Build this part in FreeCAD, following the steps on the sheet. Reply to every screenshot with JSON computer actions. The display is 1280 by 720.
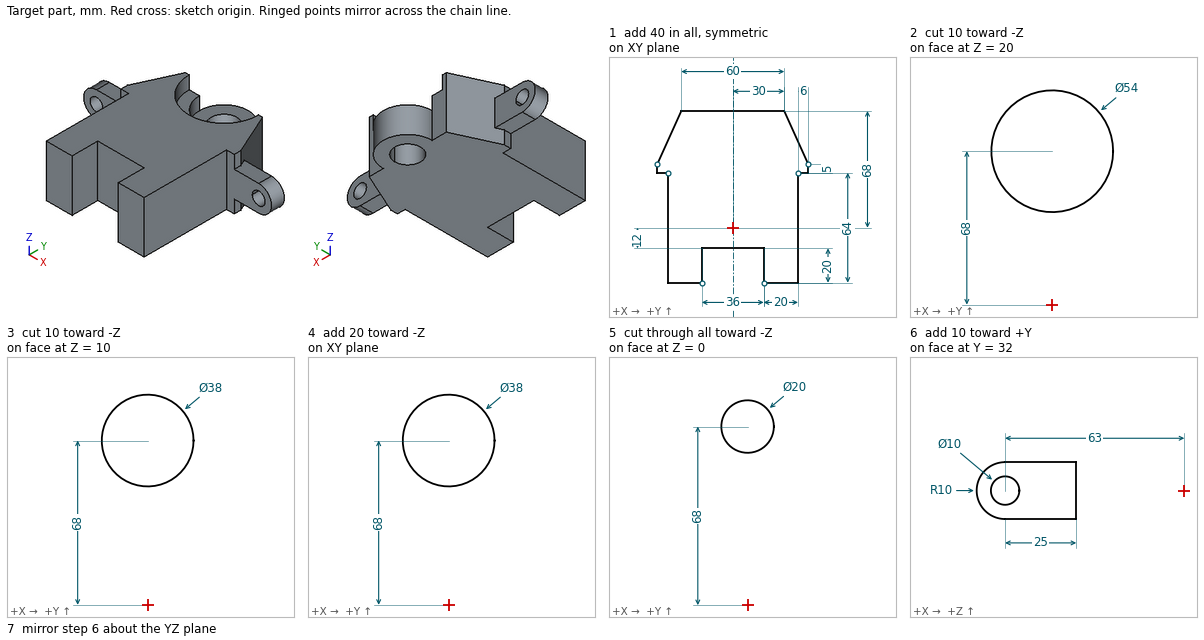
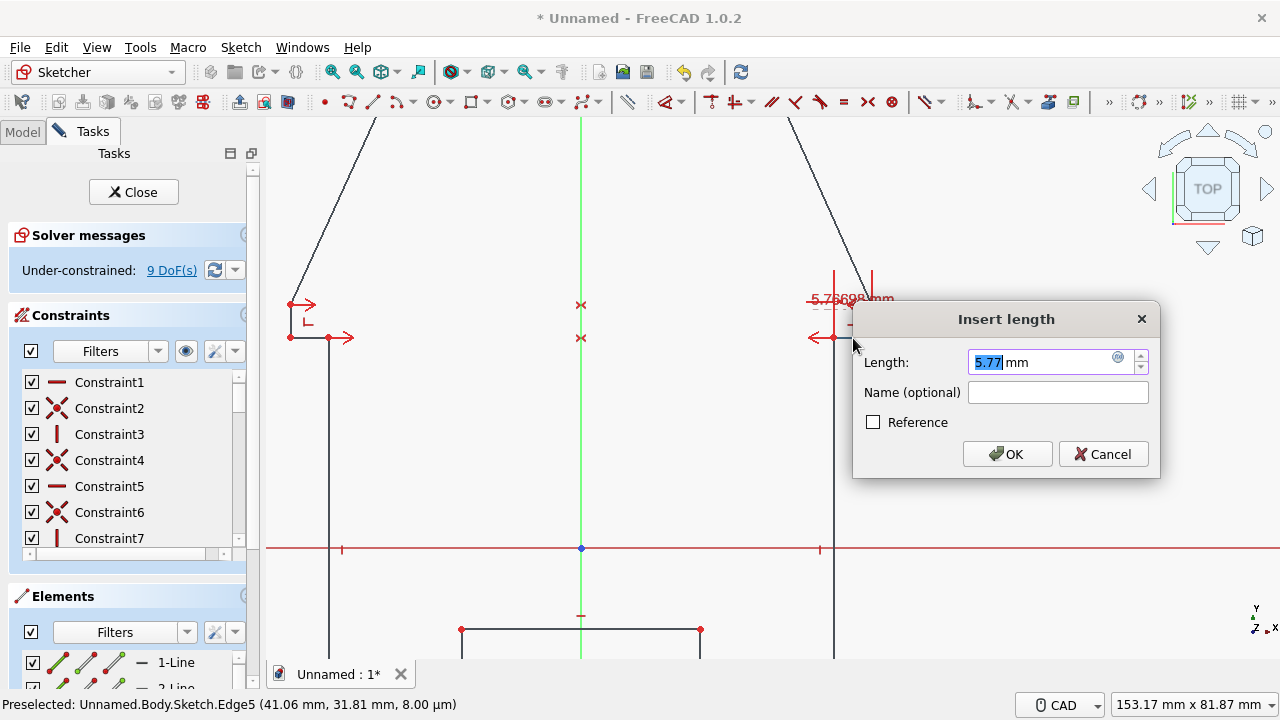
{"action": "type", "text": "6"}
{"action": "key", "text": "Return"}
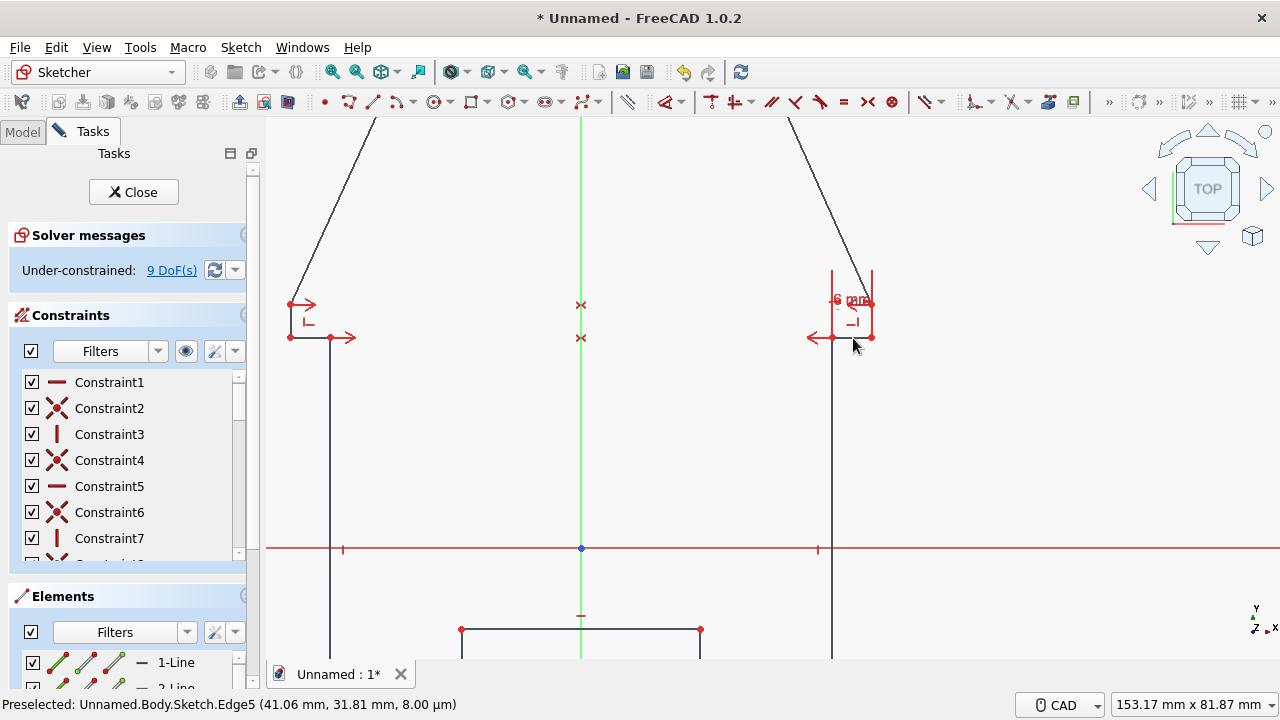
{"action": "scroll", "coordinate": [872, 328], "scroll_direction": "up", "scroll_amount": 2}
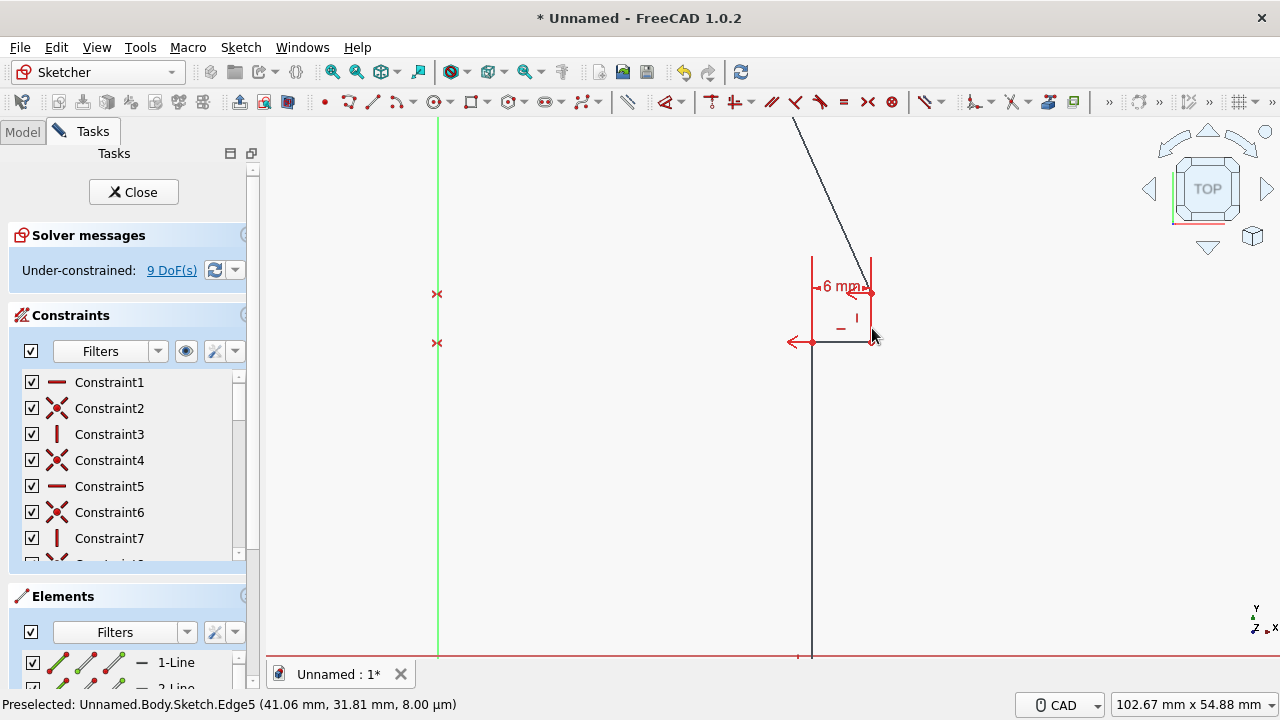
{"action": "left_click", "coordinate": [871, 328]}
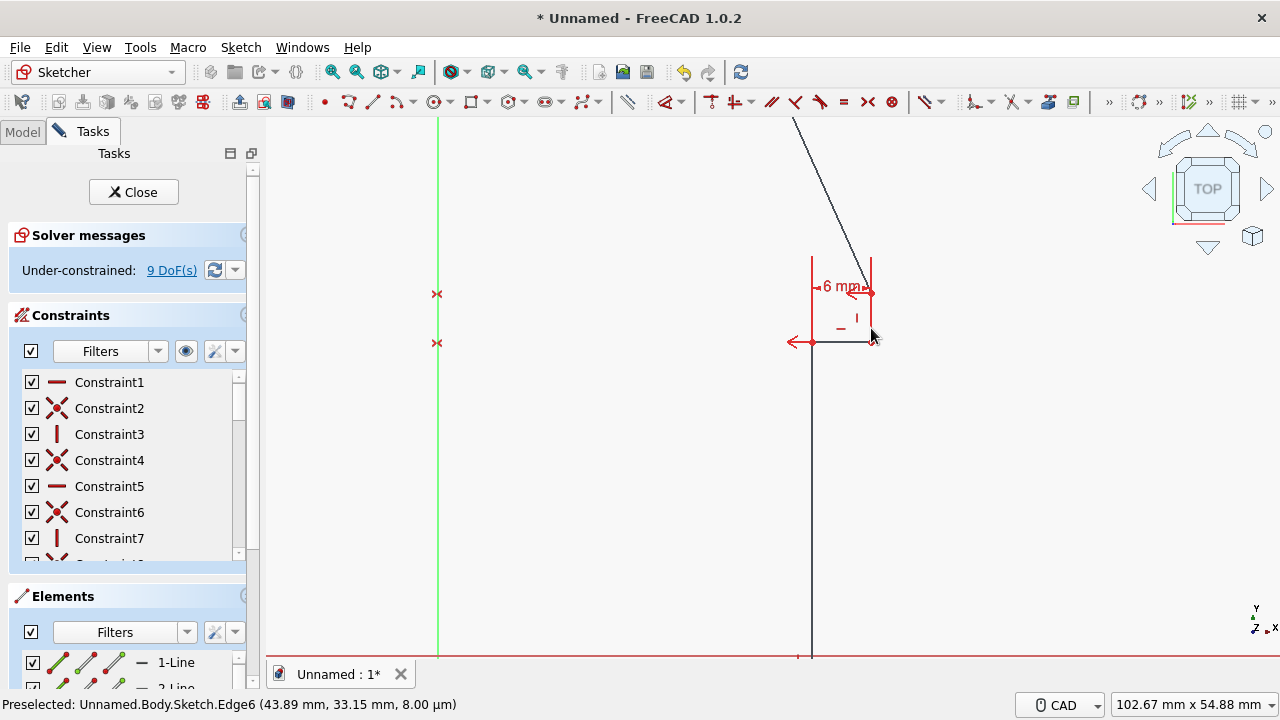
{"action": "key", "text": "i"}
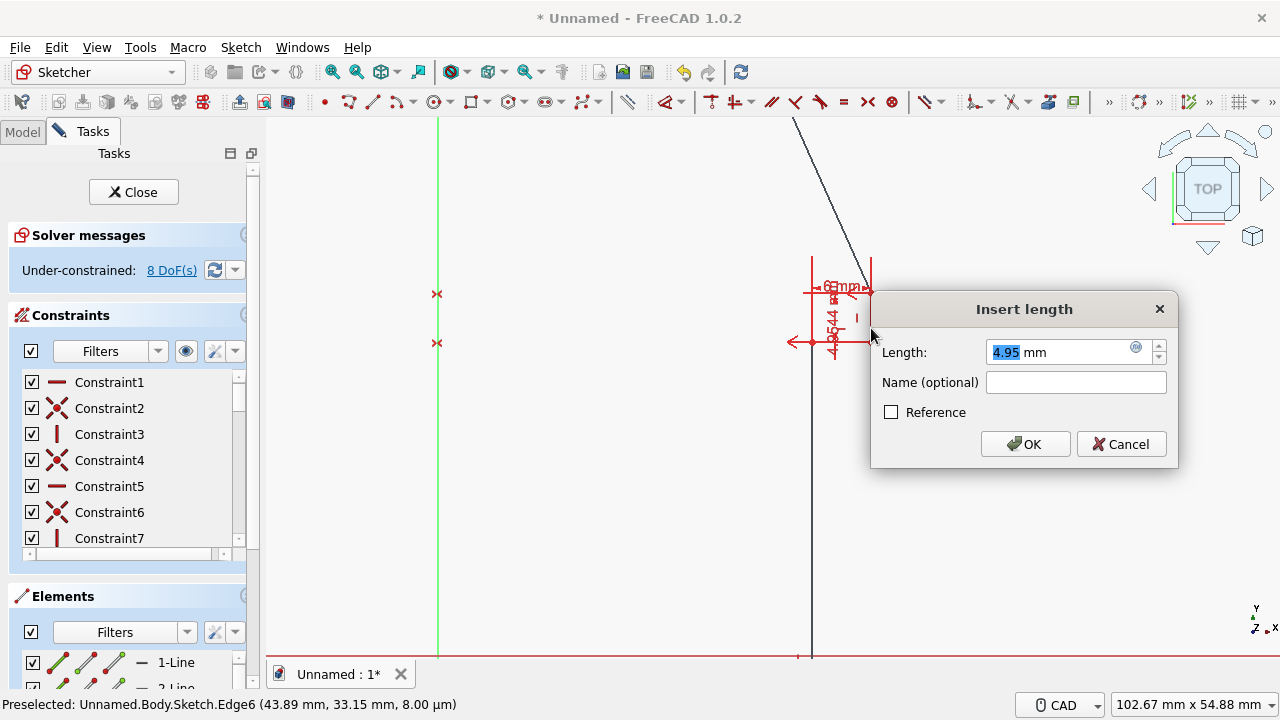
{"action": "type", "text": "5"}
{"action": "key", "text": "Return"}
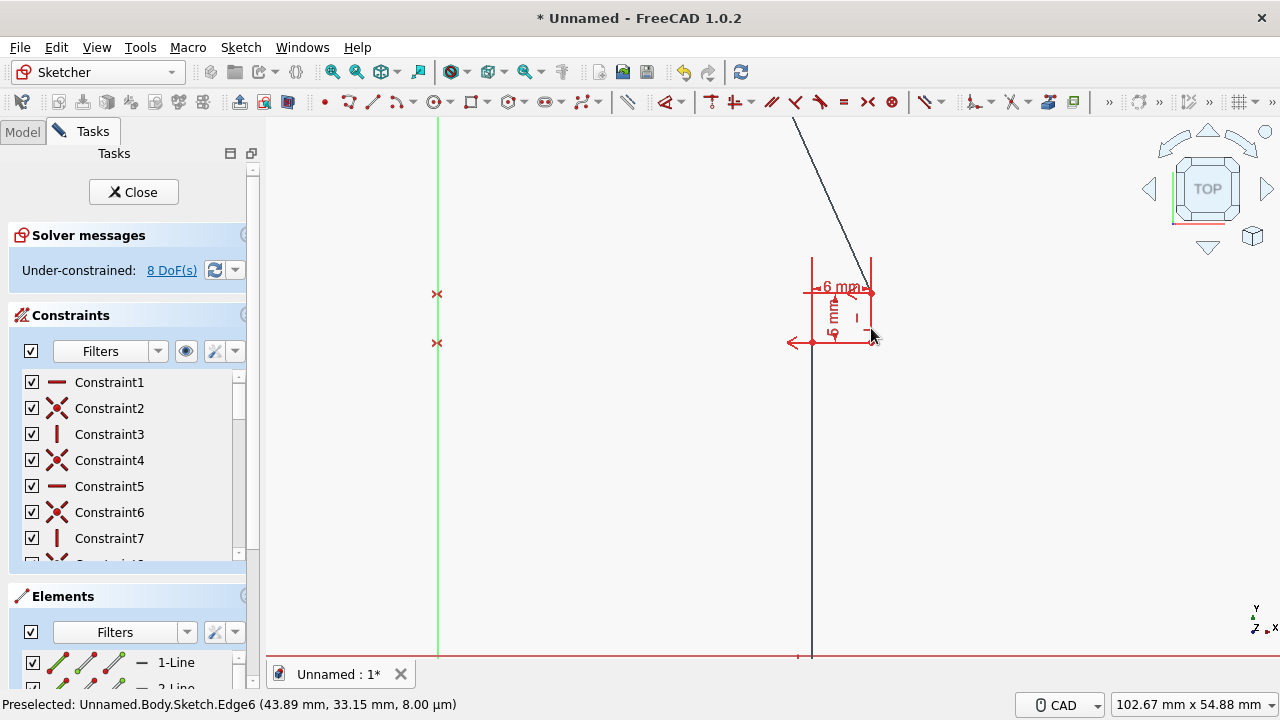
{"action": "scroll", "coordinate": [860, 335], "scroll_direction": "down", "scroll_amount": 5}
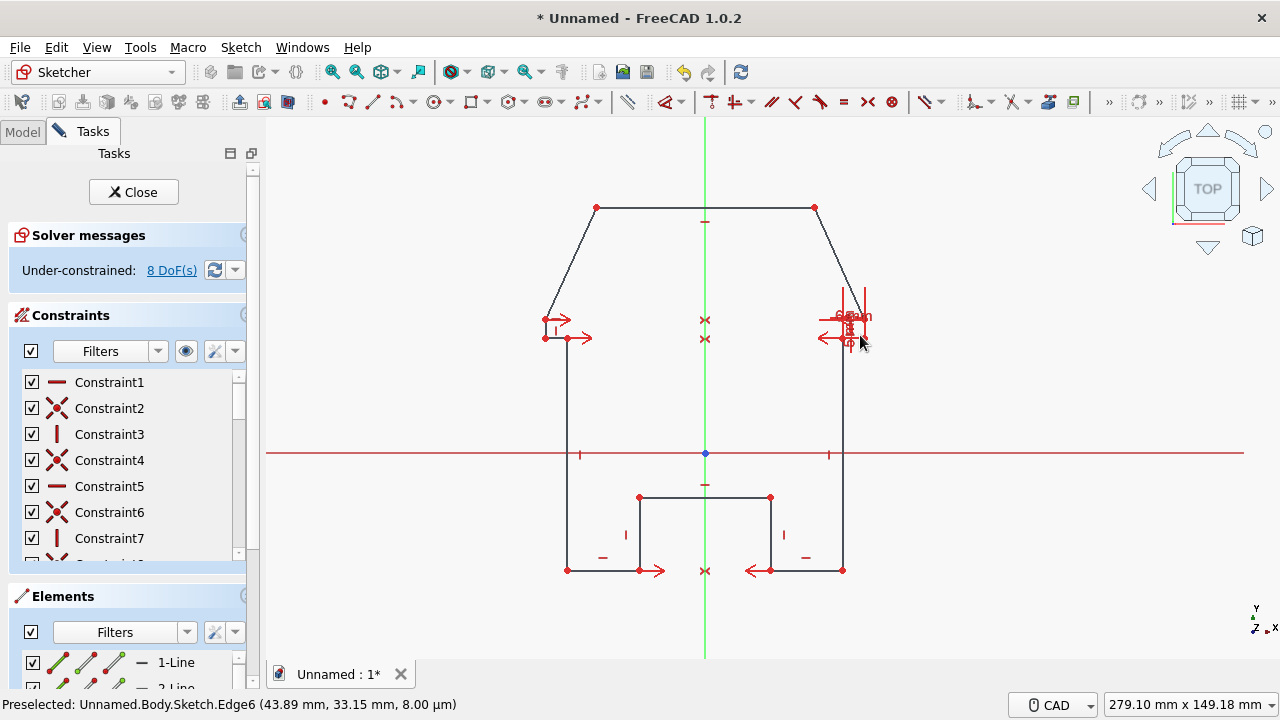
{"action": "left_click", "coordinate": [679, 498]}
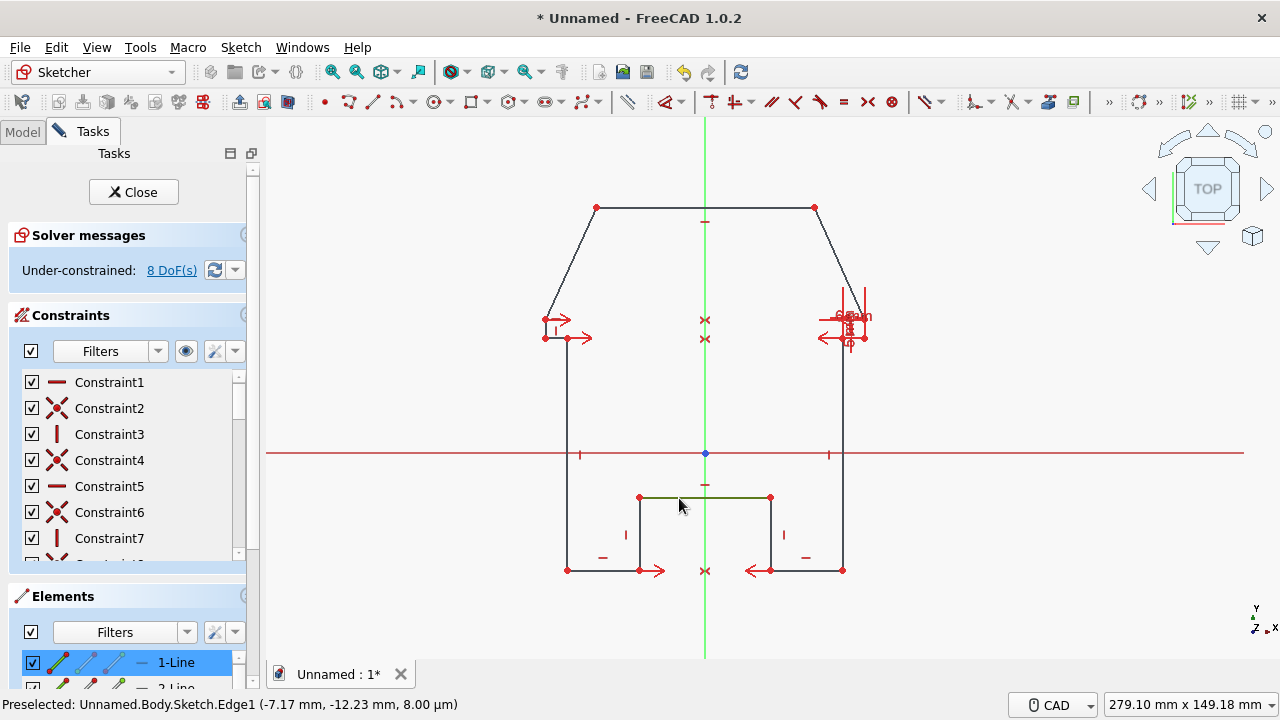
{"action": "left_click", "coordinate": [684, 102]}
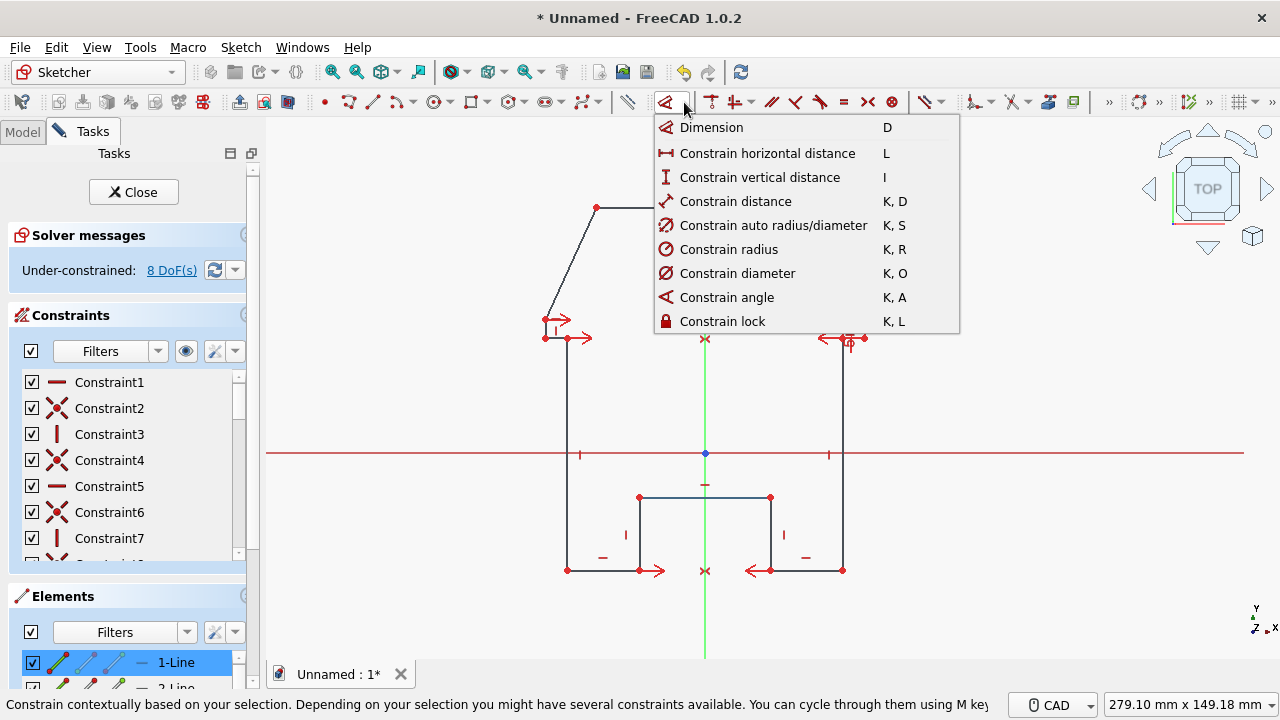
{"action": "left_click", "coordinate": [807, 153]}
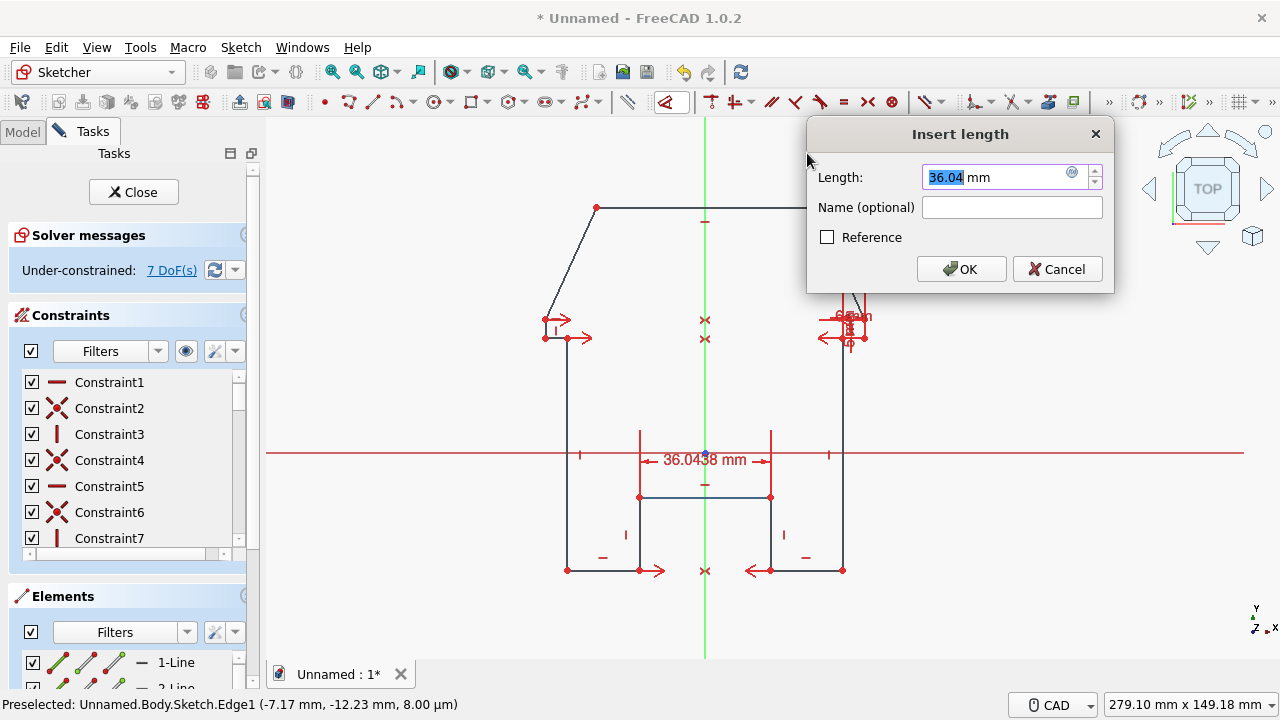
{"action": "type", "text": "36"}
{"action": "key", "text": "Return"}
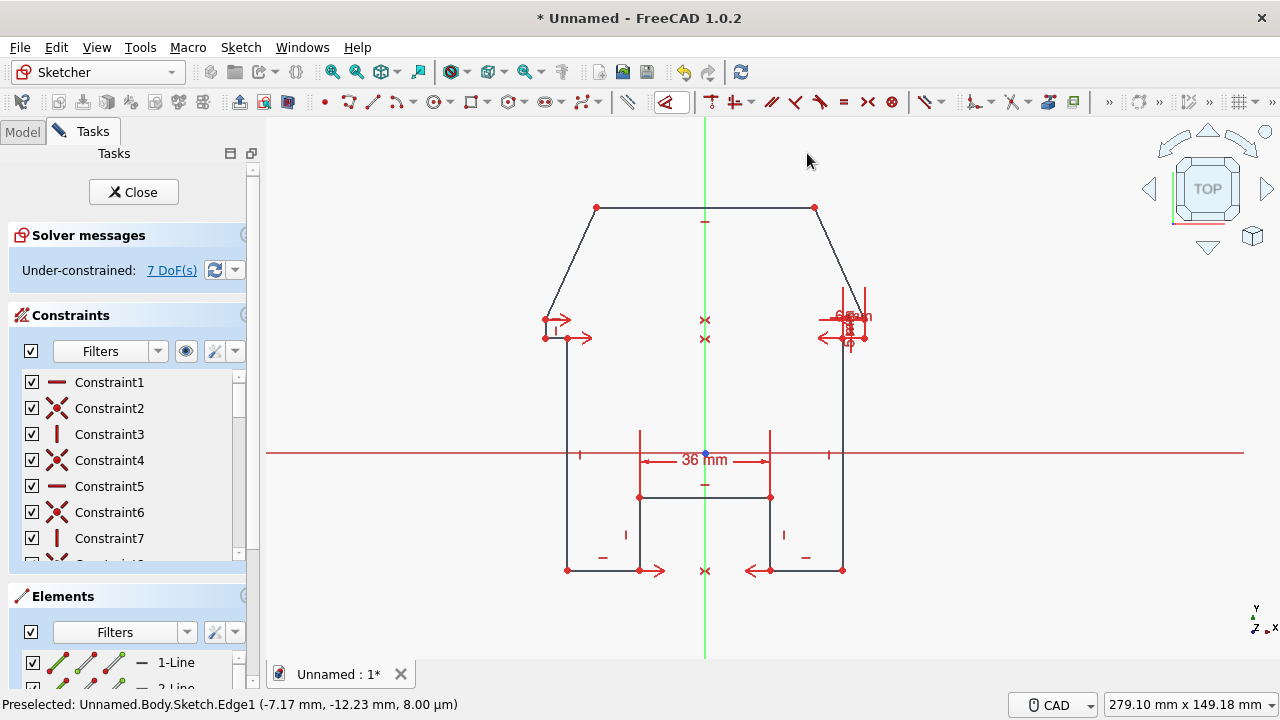
{"action": "left_click", "coordinate": [770, 520]}